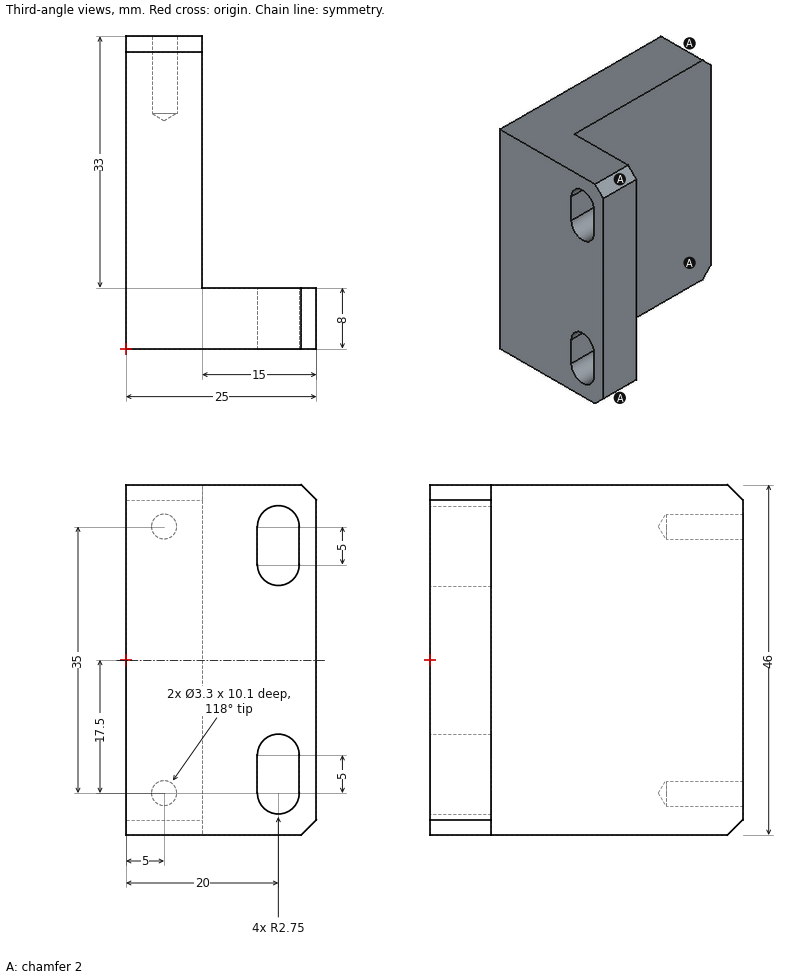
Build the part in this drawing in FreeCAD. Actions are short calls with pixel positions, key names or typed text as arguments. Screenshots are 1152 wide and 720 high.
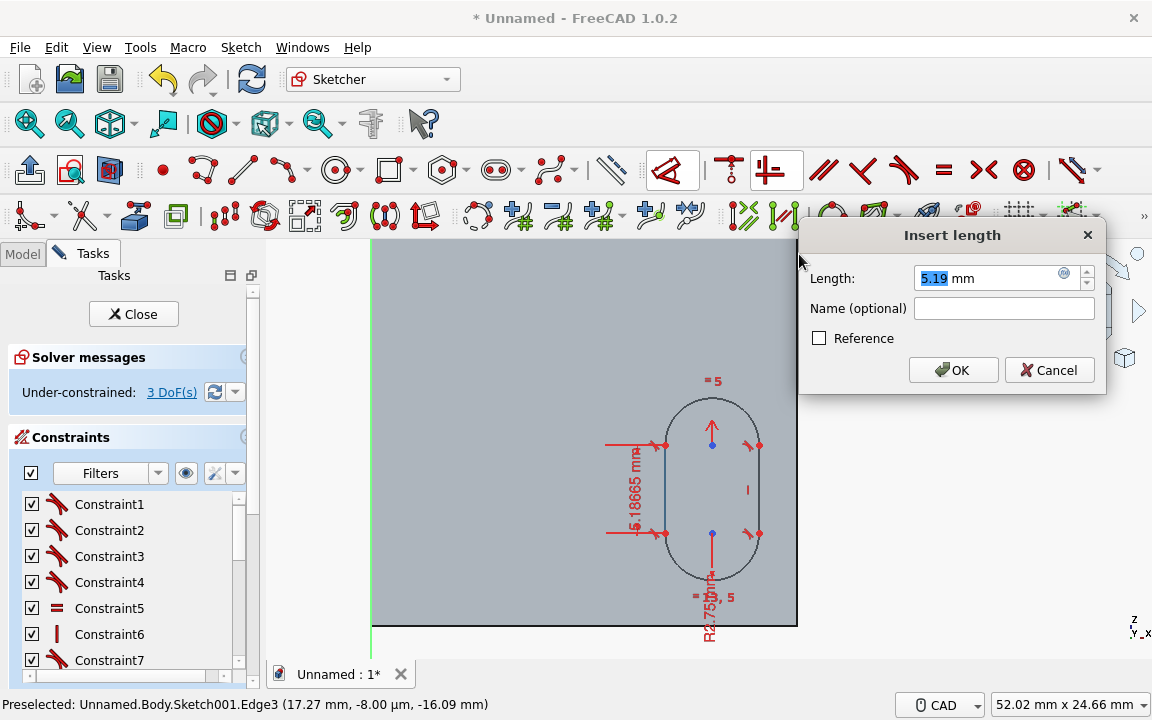
text(5)
key(Return)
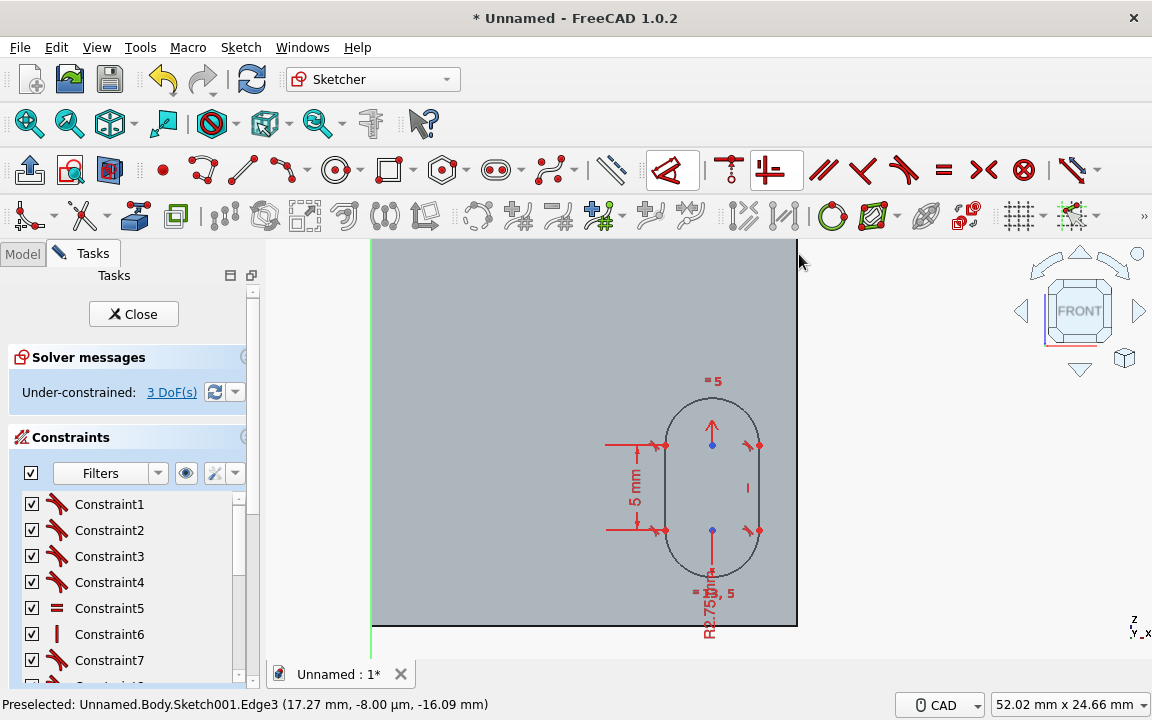
scroll(684, 574, down, 5)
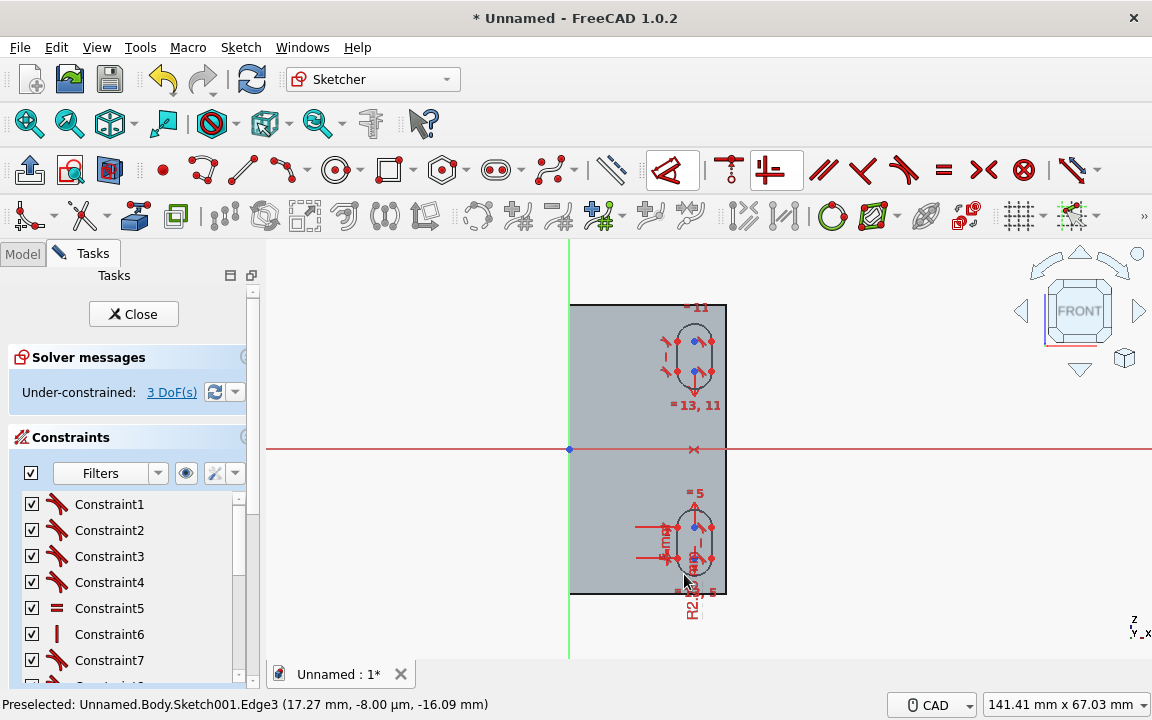
scroll(677, 363, up, 3)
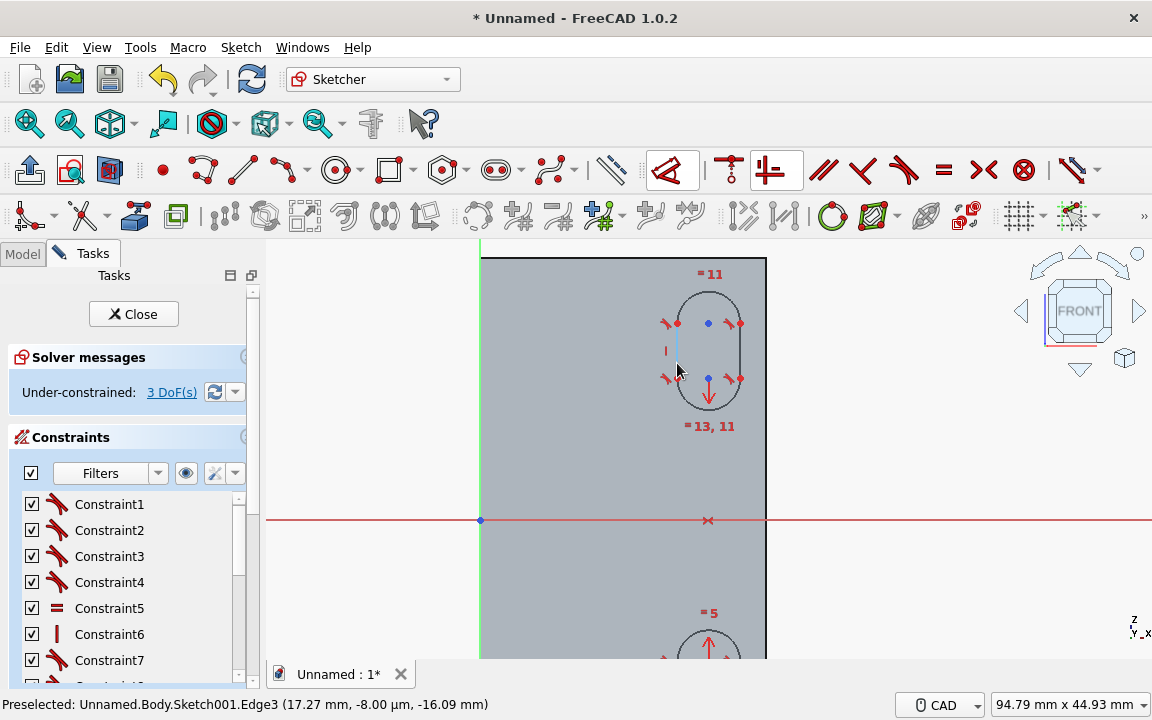
click(677, 362)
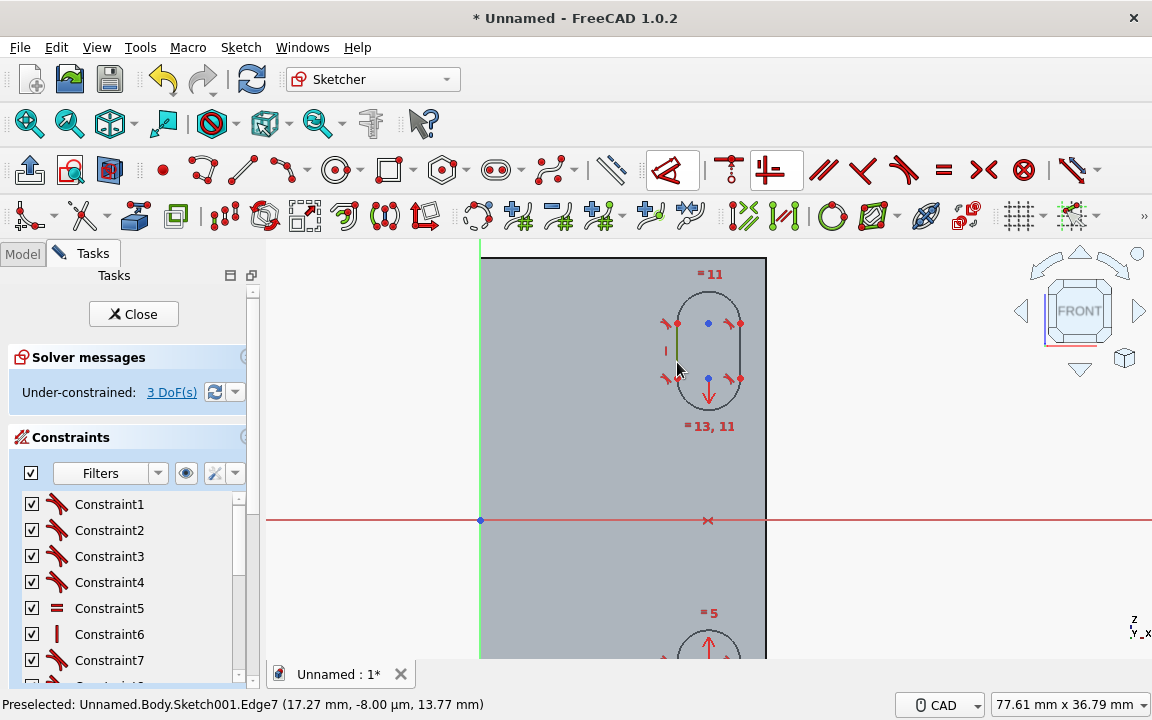
click(694, 170)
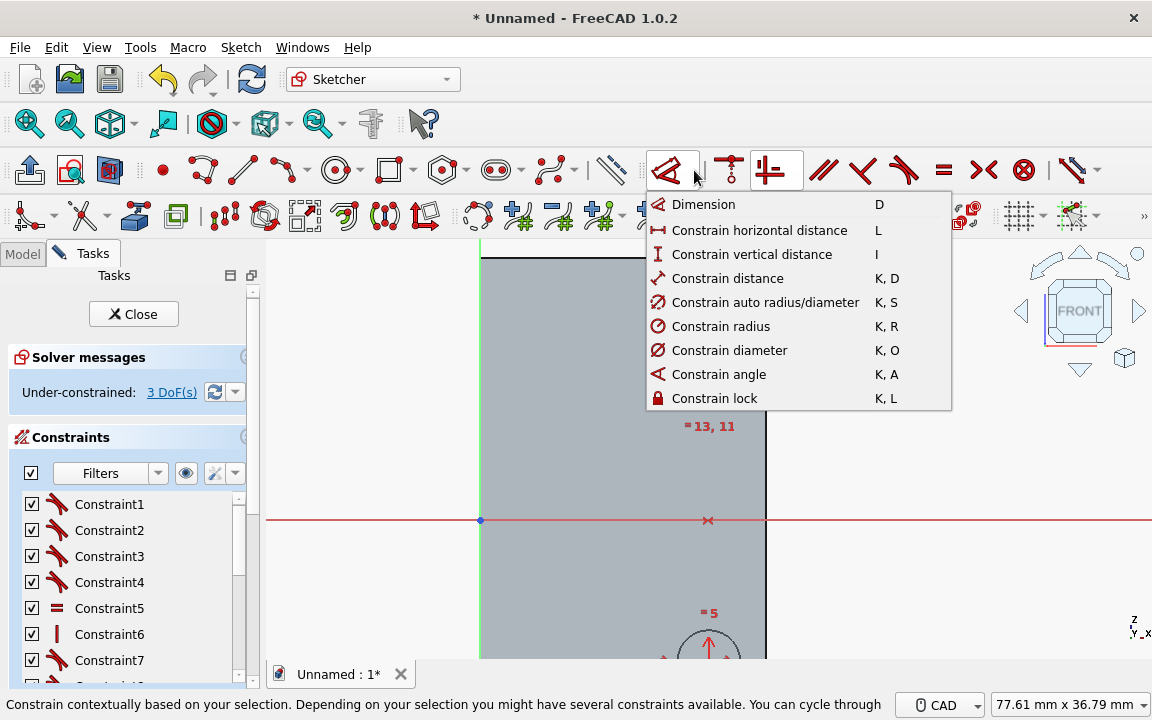
click(799, 254)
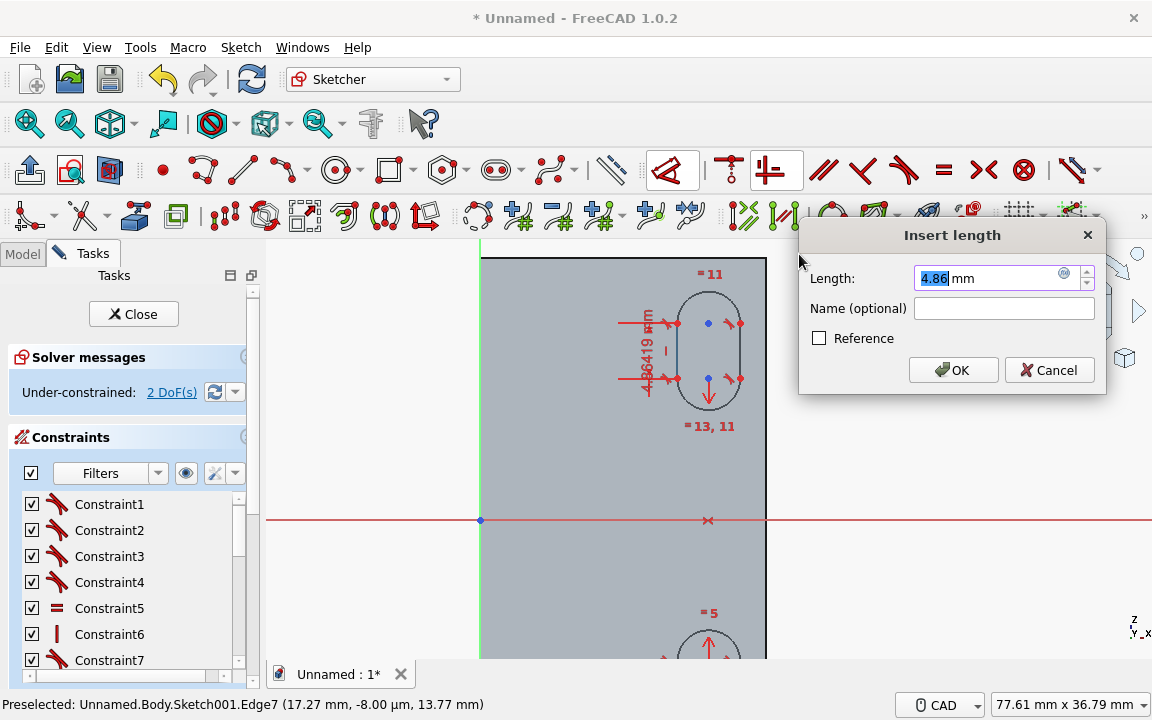
text(5)
key(Return)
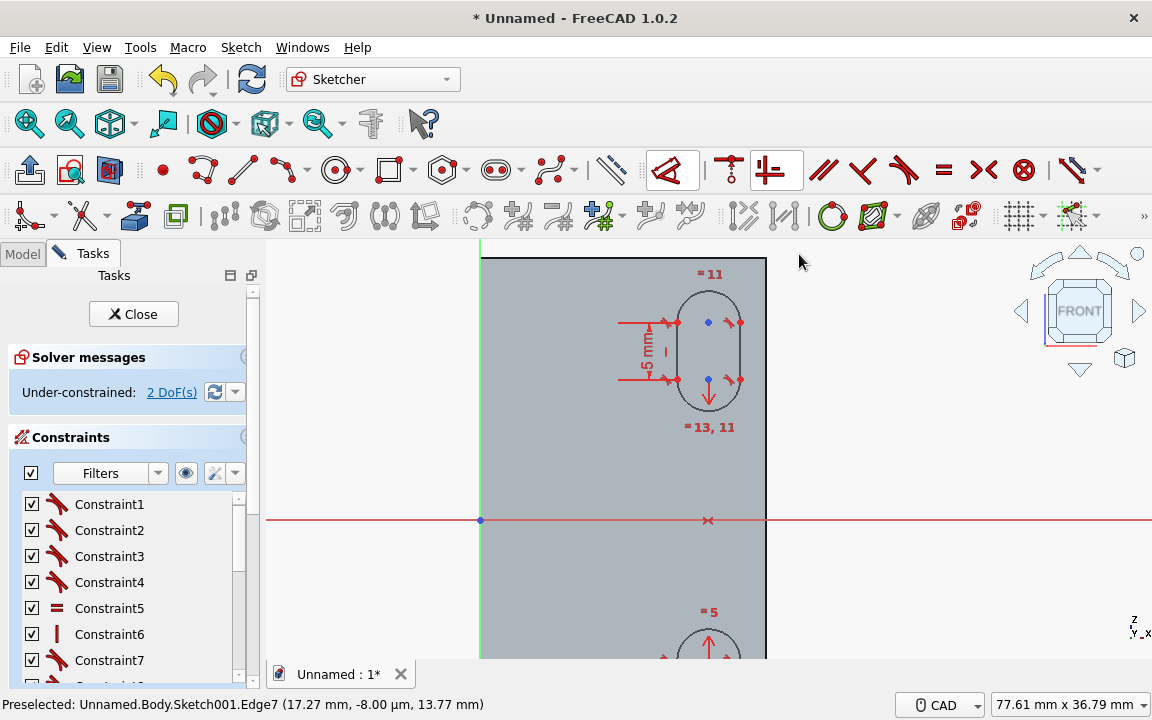
scroll(677, 362, down, 3)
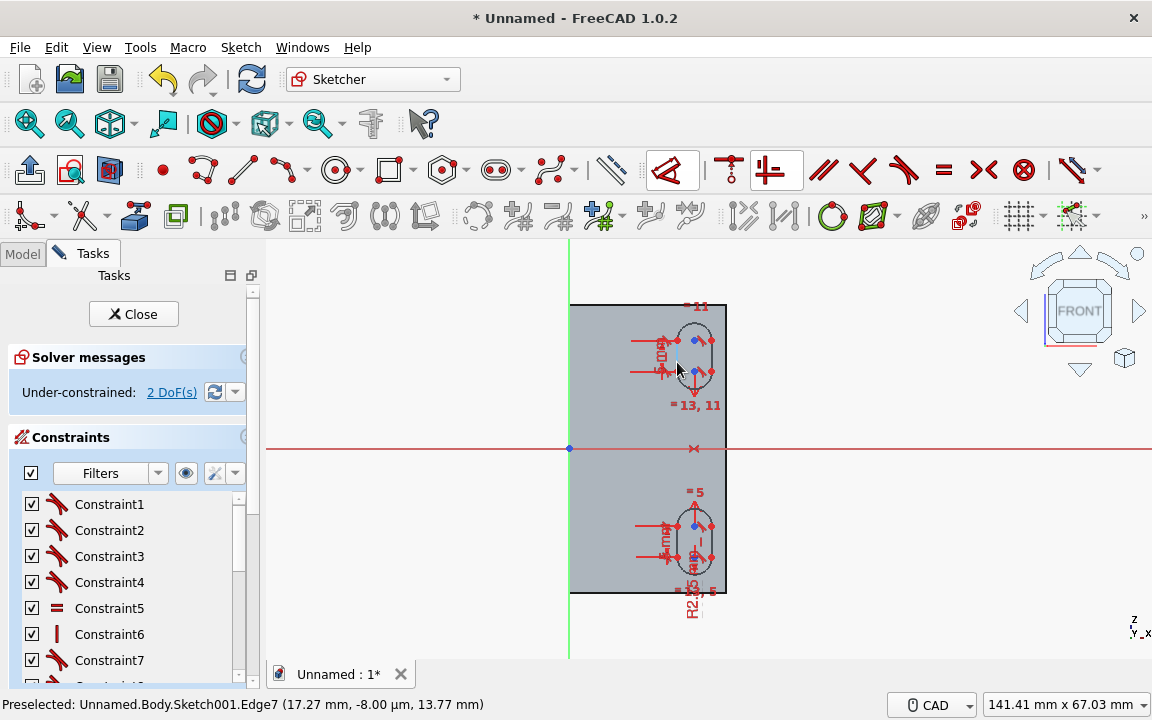
click(695, 557)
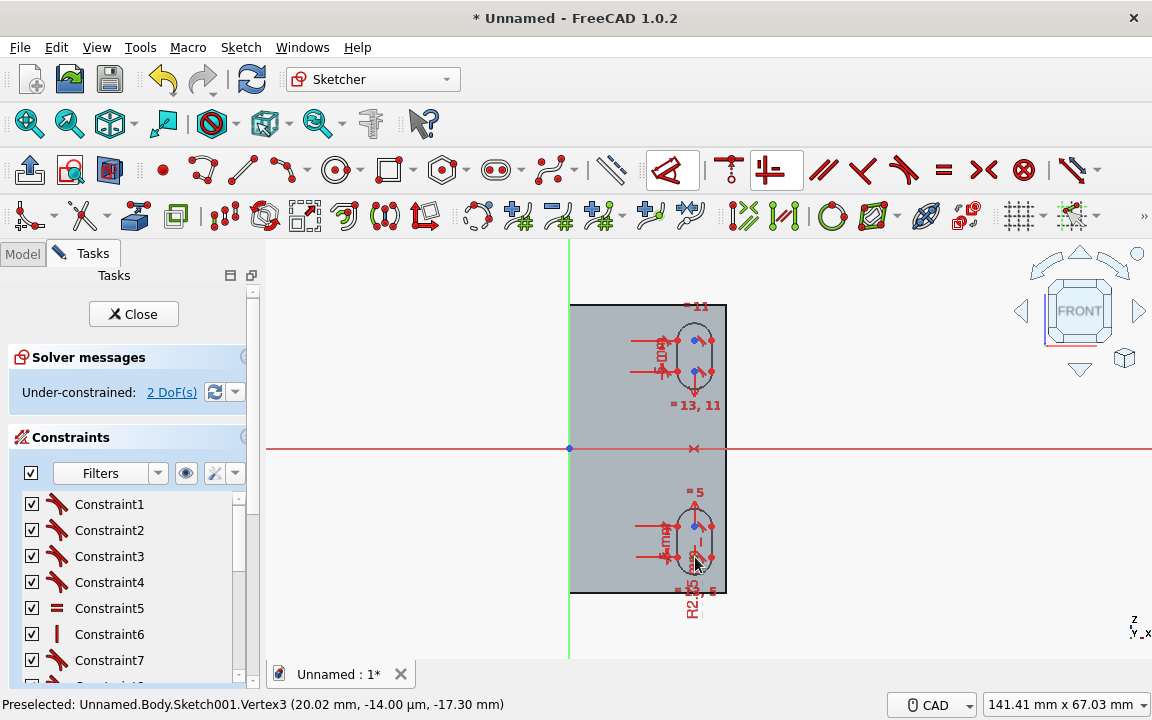
click(694, 170)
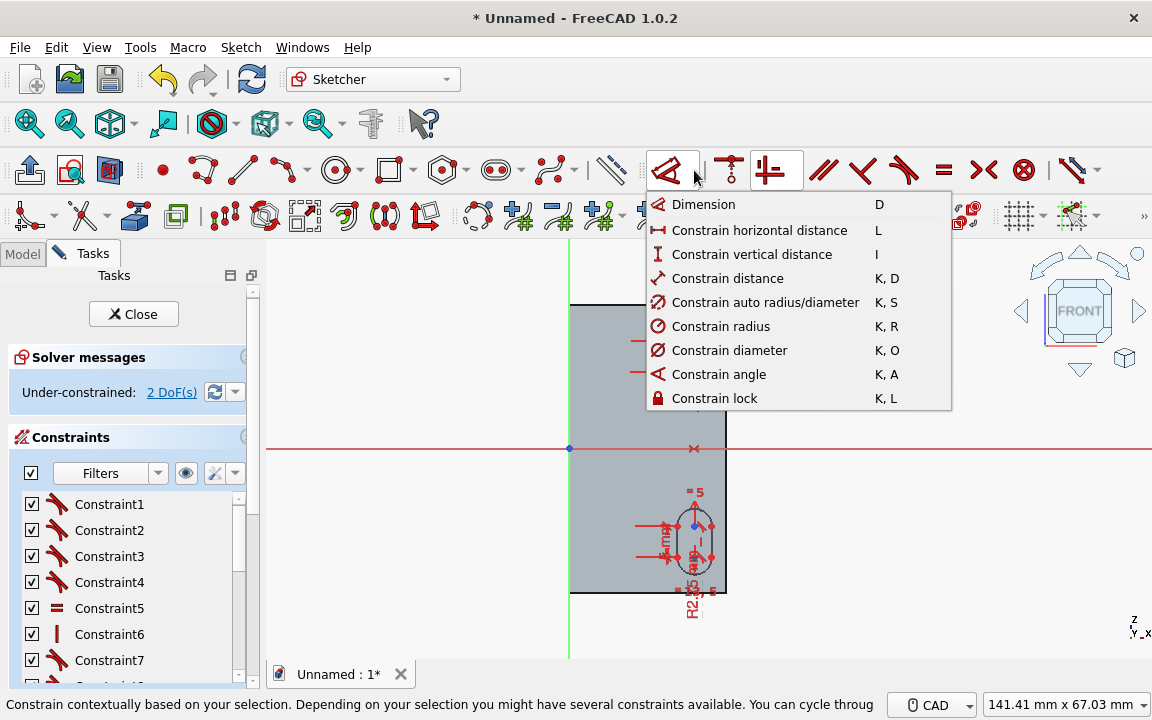
click(799, 230)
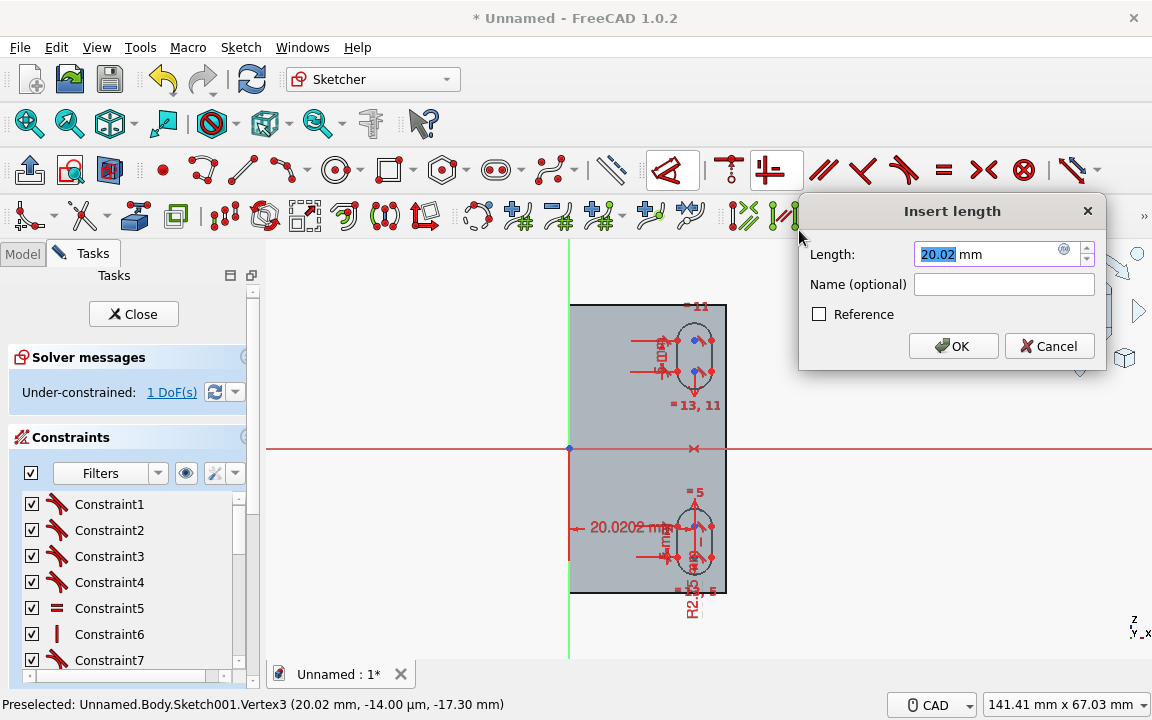
text(20)
key(Return)